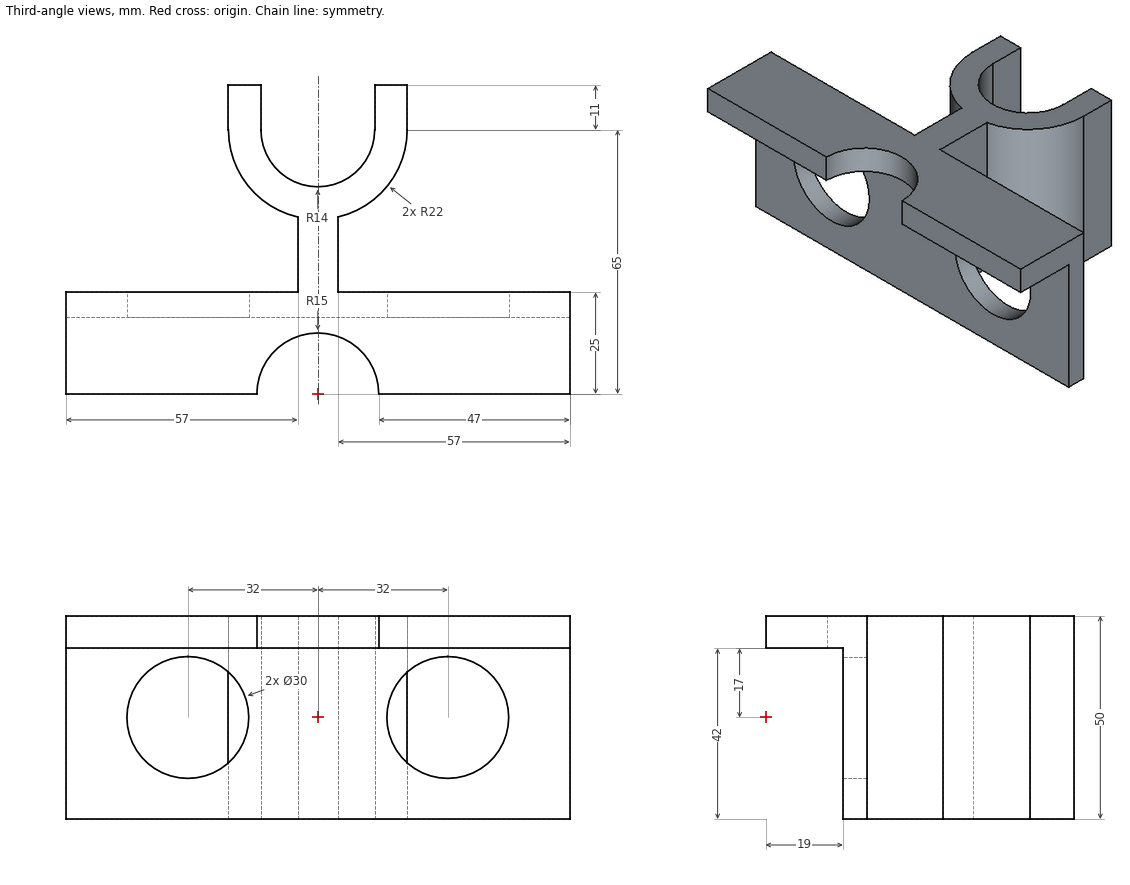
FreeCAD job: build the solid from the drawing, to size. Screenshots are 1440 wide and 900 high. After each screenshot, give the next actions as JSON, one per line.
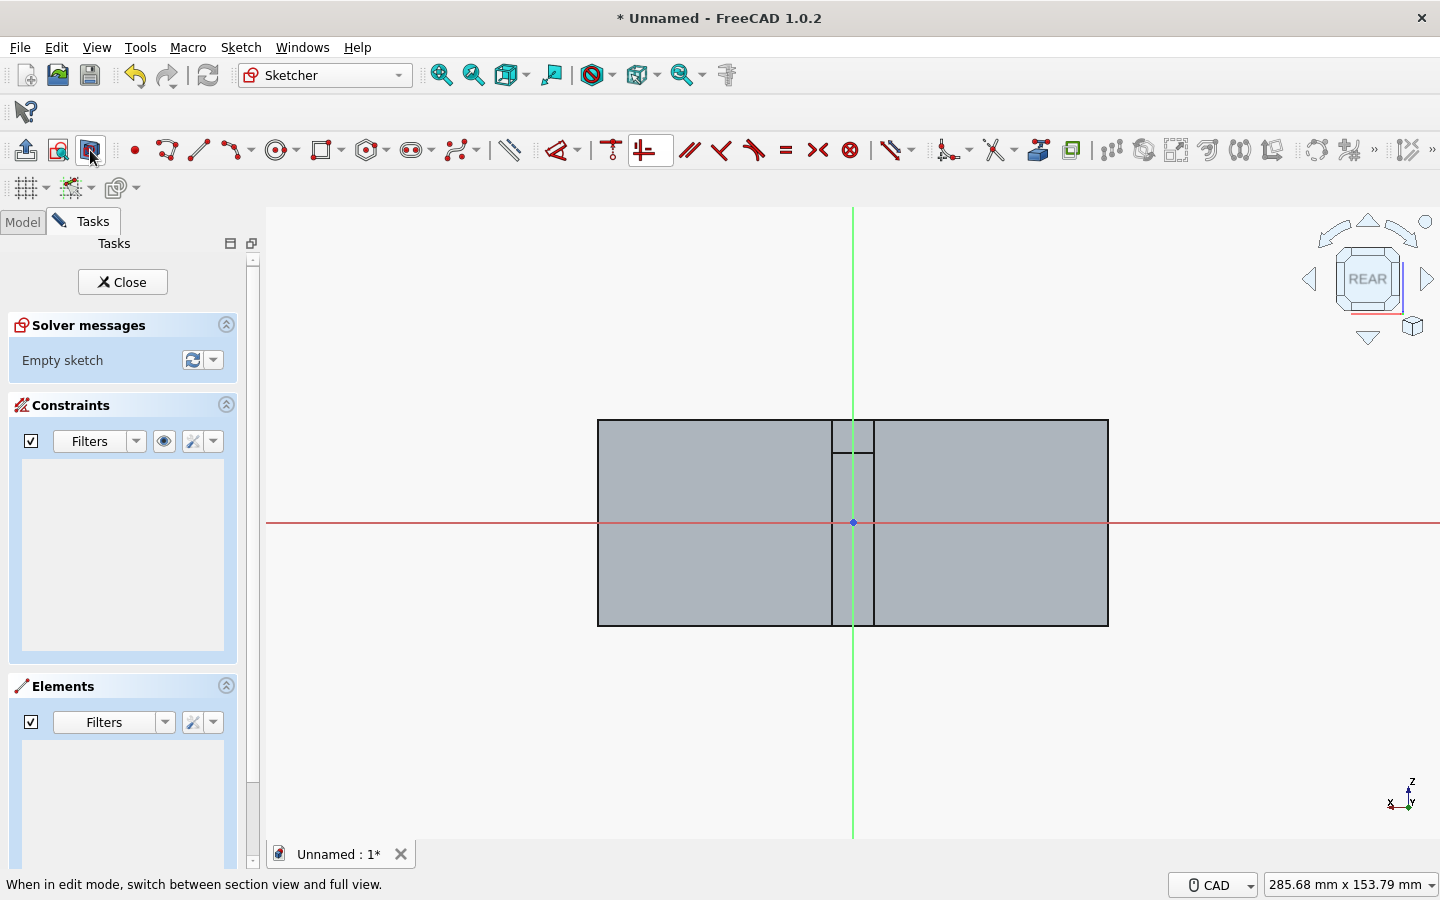
{"action": "scroll", "coordinate": [936, 523], "scroll_direction": "up", "scroll_amount": 3}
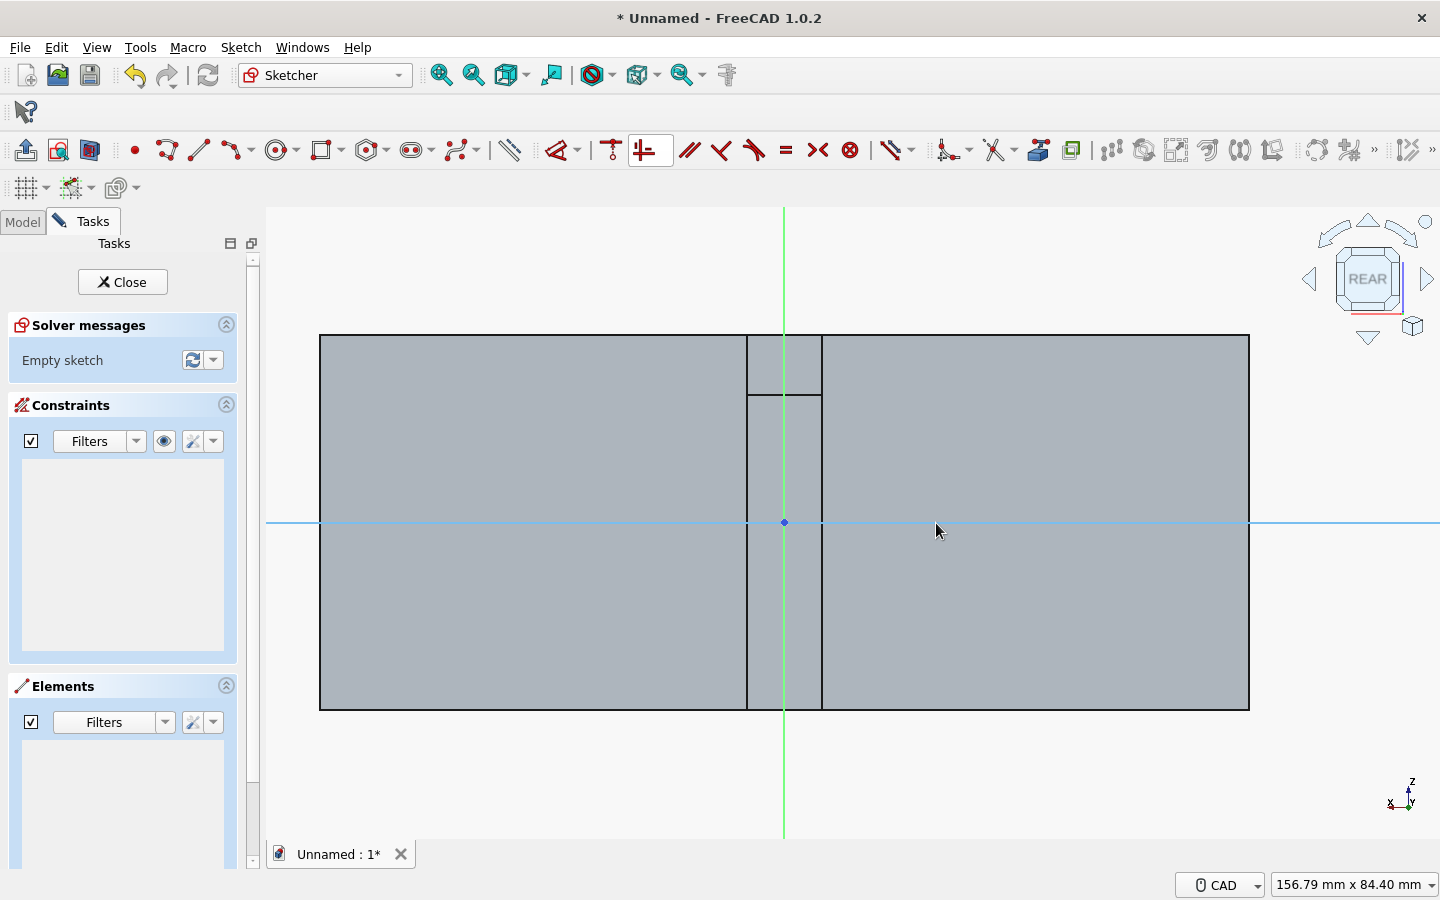
{"action": "left_click", "coordinate": [276, 150]}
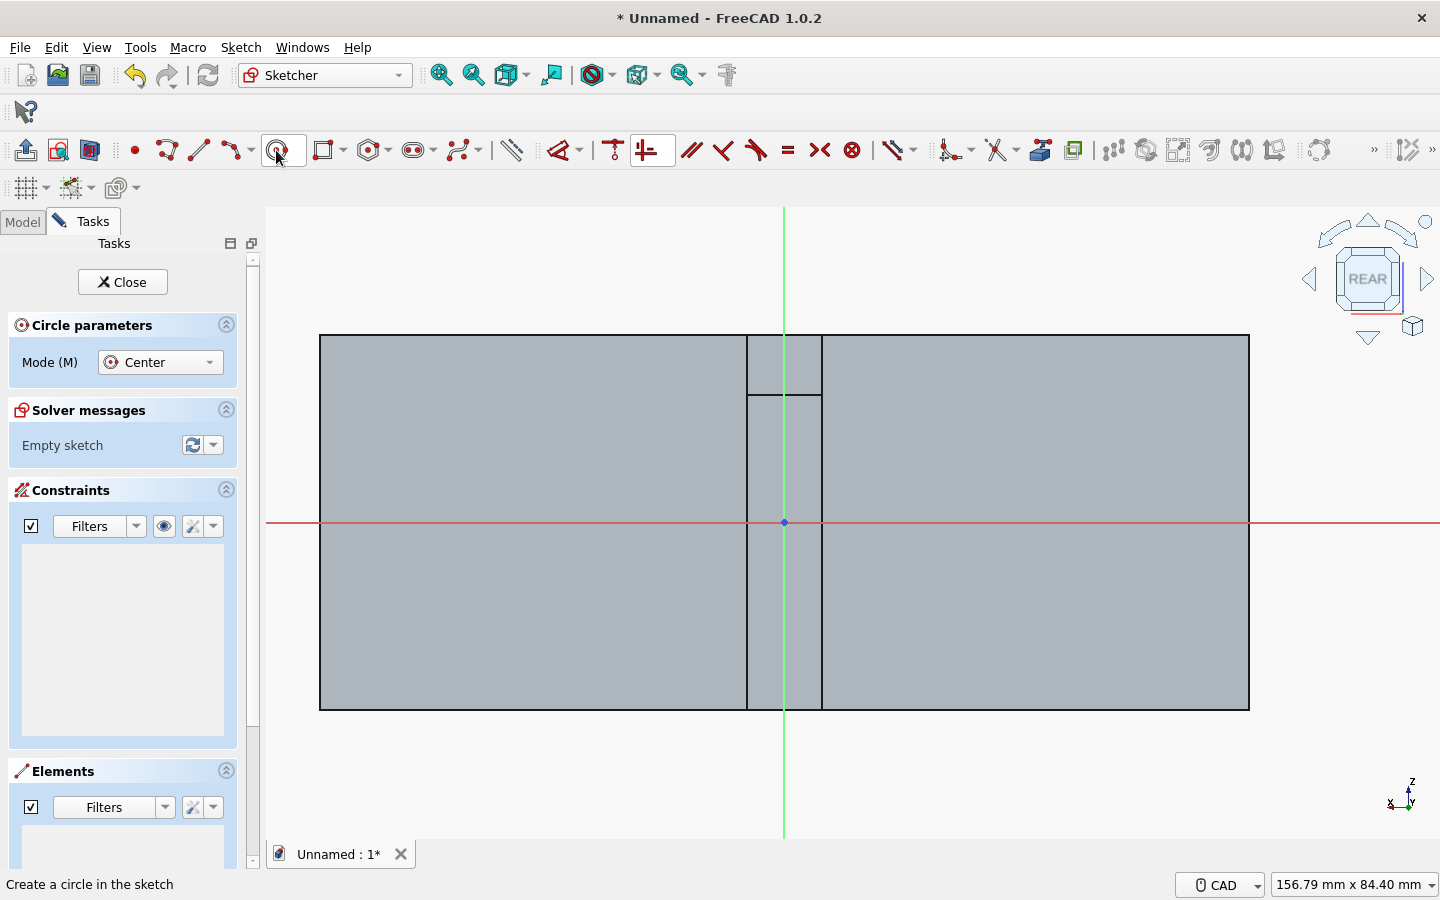
{"action": "left_click", "coordinate": [1024, 523]}
{"action": "left_click", "coordinate": [1103, 443]}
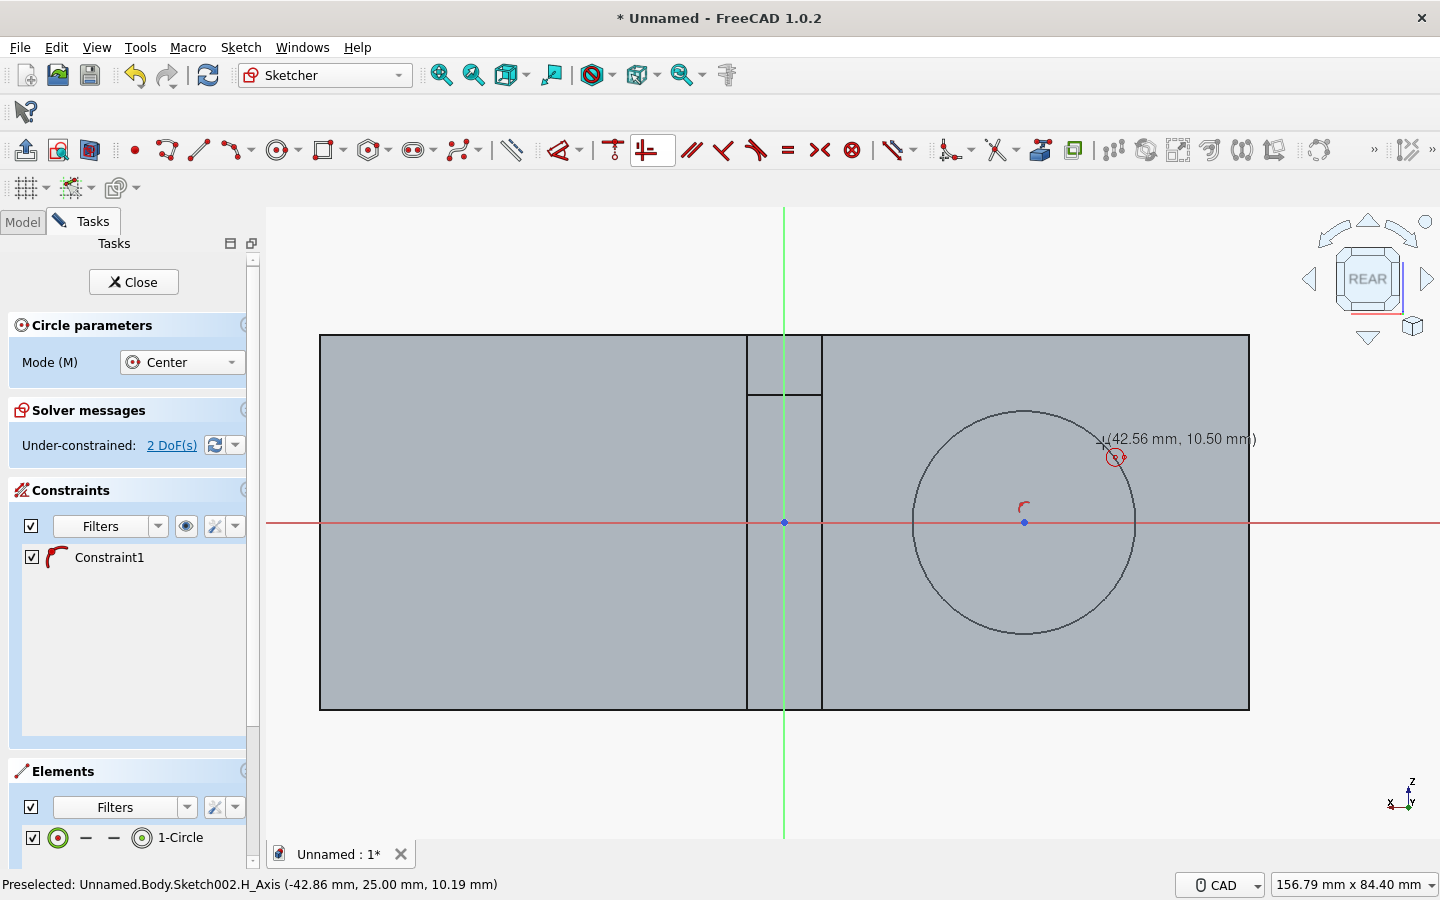
{"action": "left_click", "coordinate": [545, 523]}
{"action": "left_click", "coordinate": [624, 443]}
{"action": "key", "text": "Escape"}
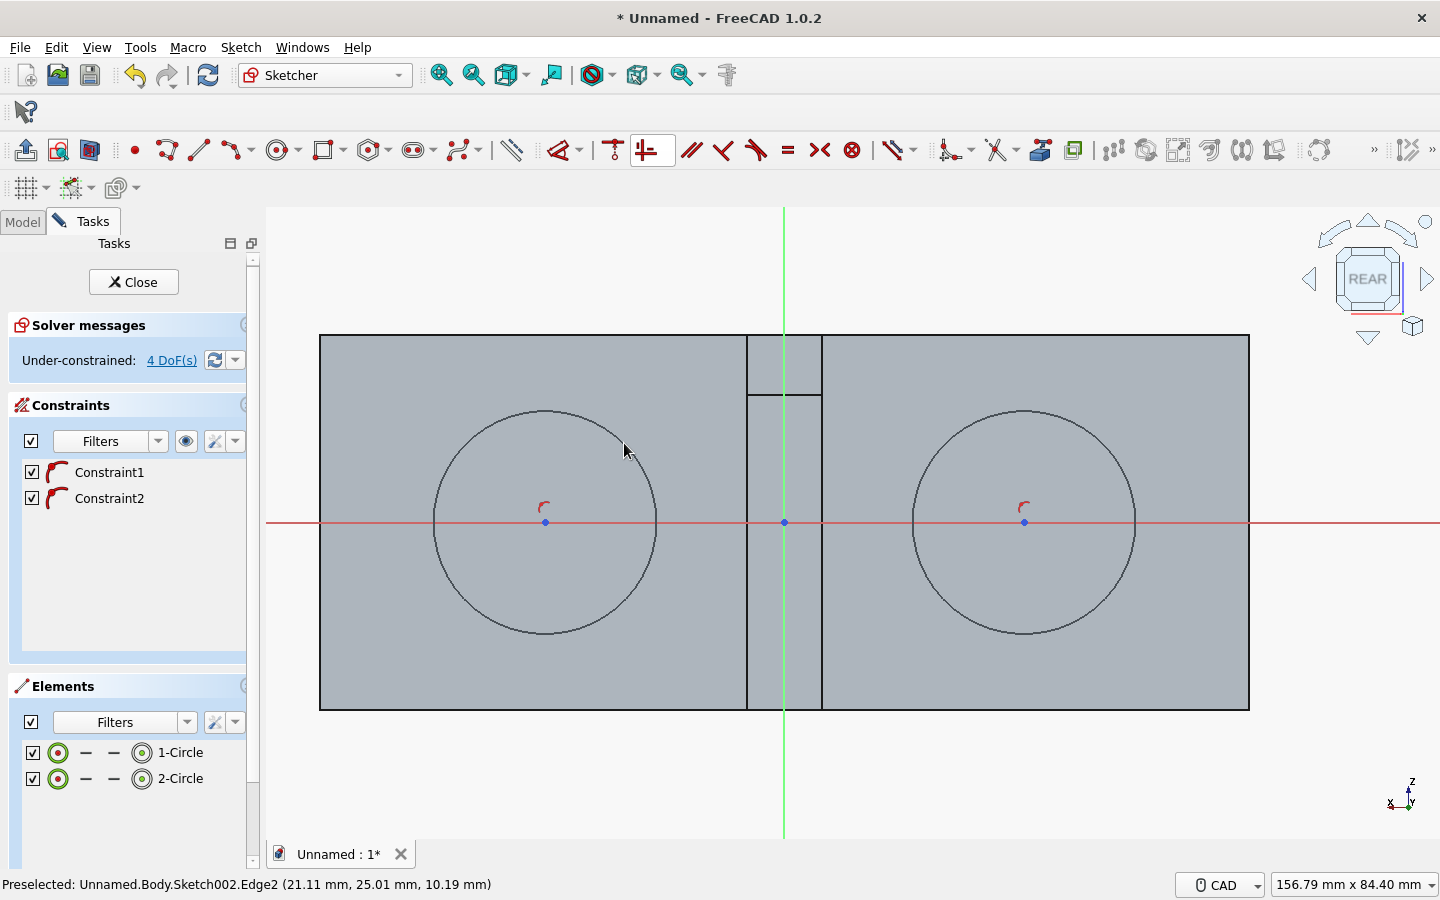
{"action": "left_click", "coordinate": [1103, 444]}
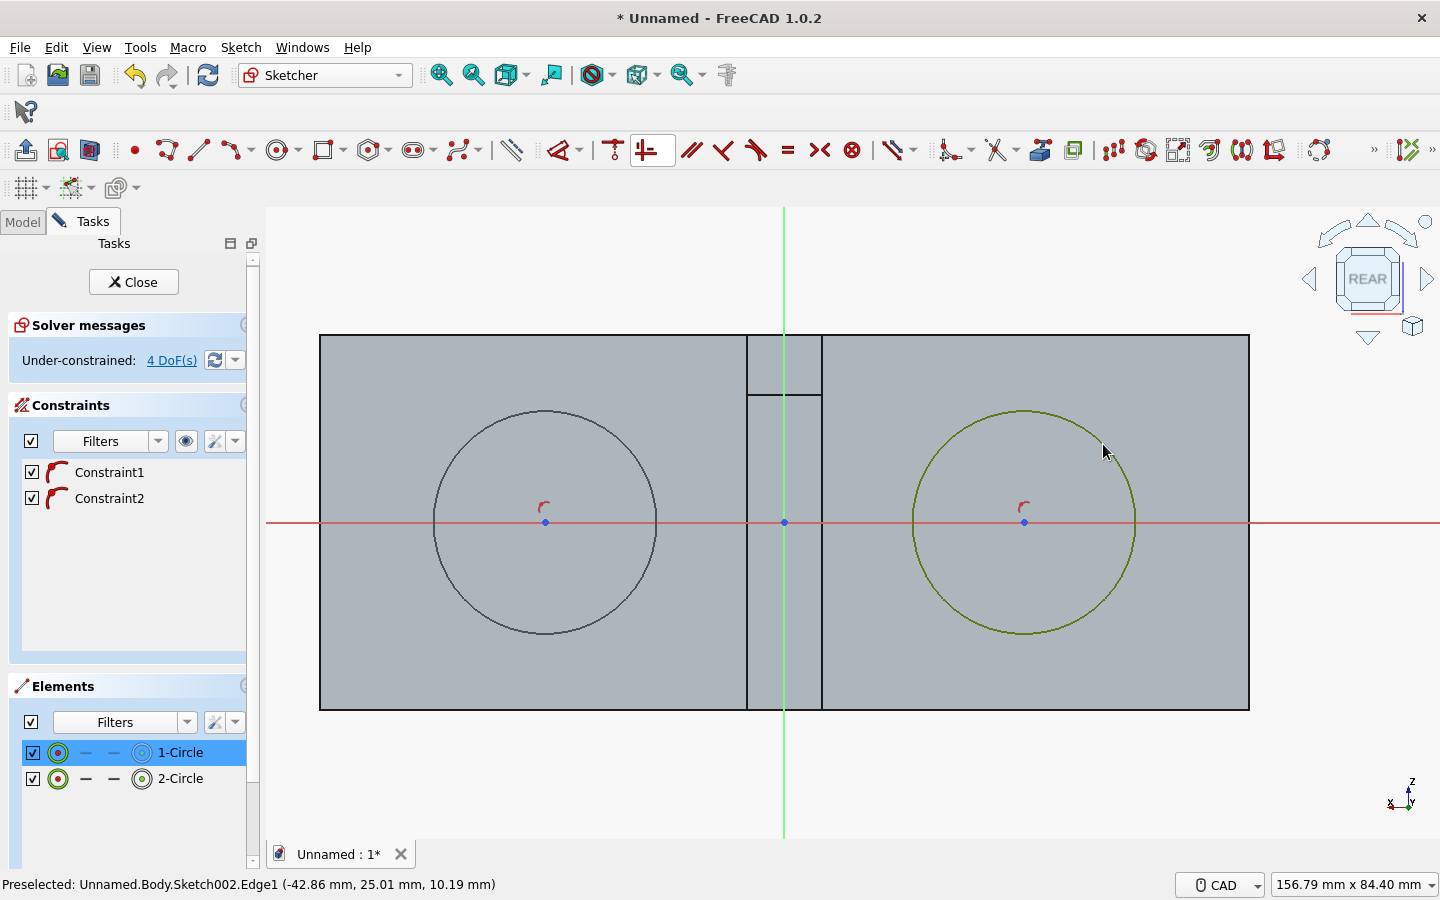
{"action": "left_click", "coordinate": [624, 444]}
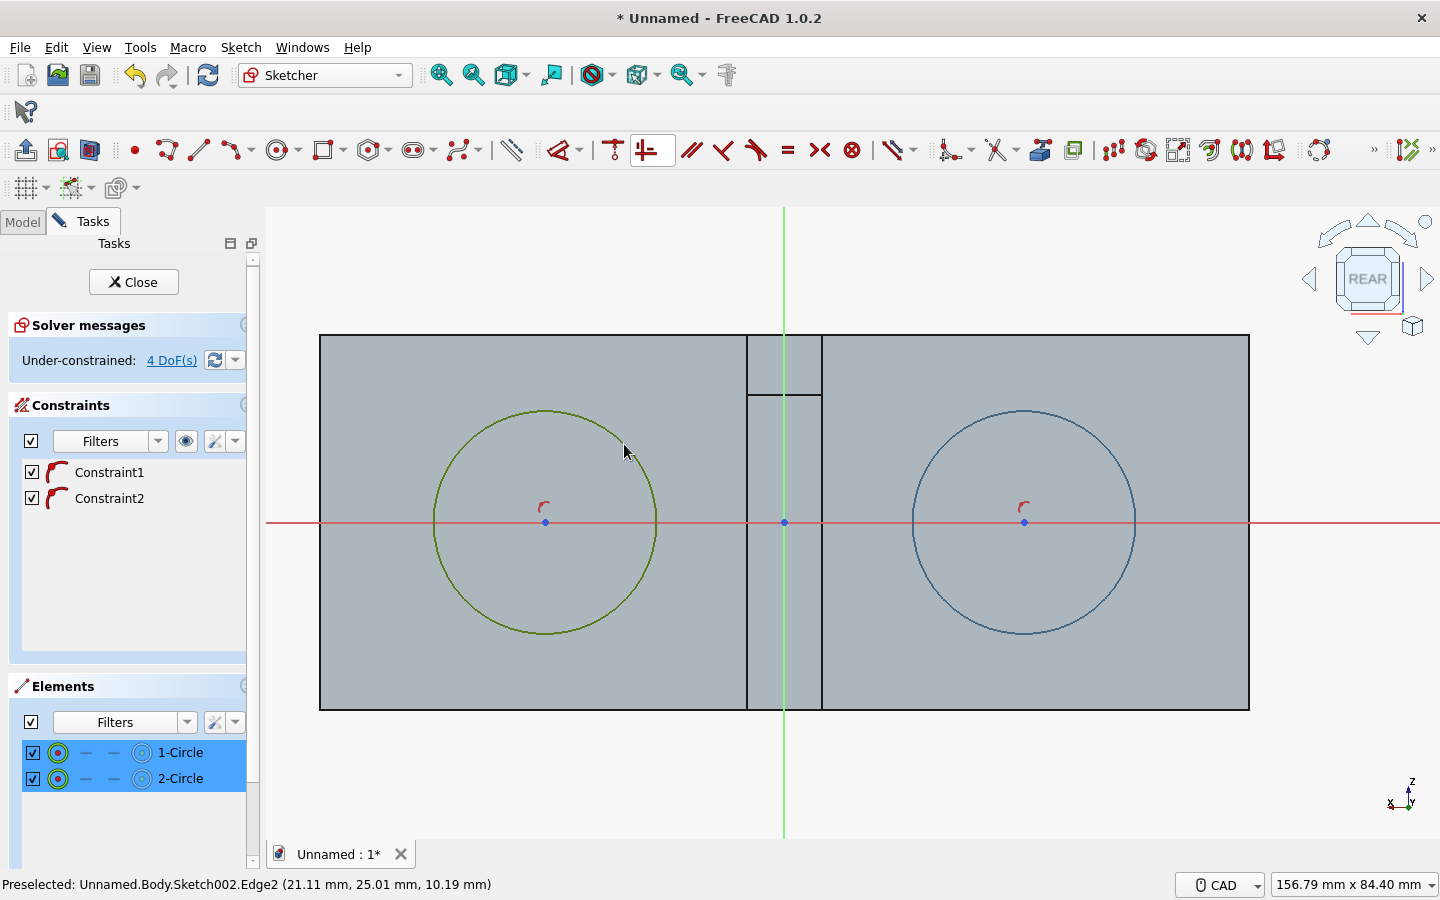
{"action": "left_click", "coordinate": [788, 150]}